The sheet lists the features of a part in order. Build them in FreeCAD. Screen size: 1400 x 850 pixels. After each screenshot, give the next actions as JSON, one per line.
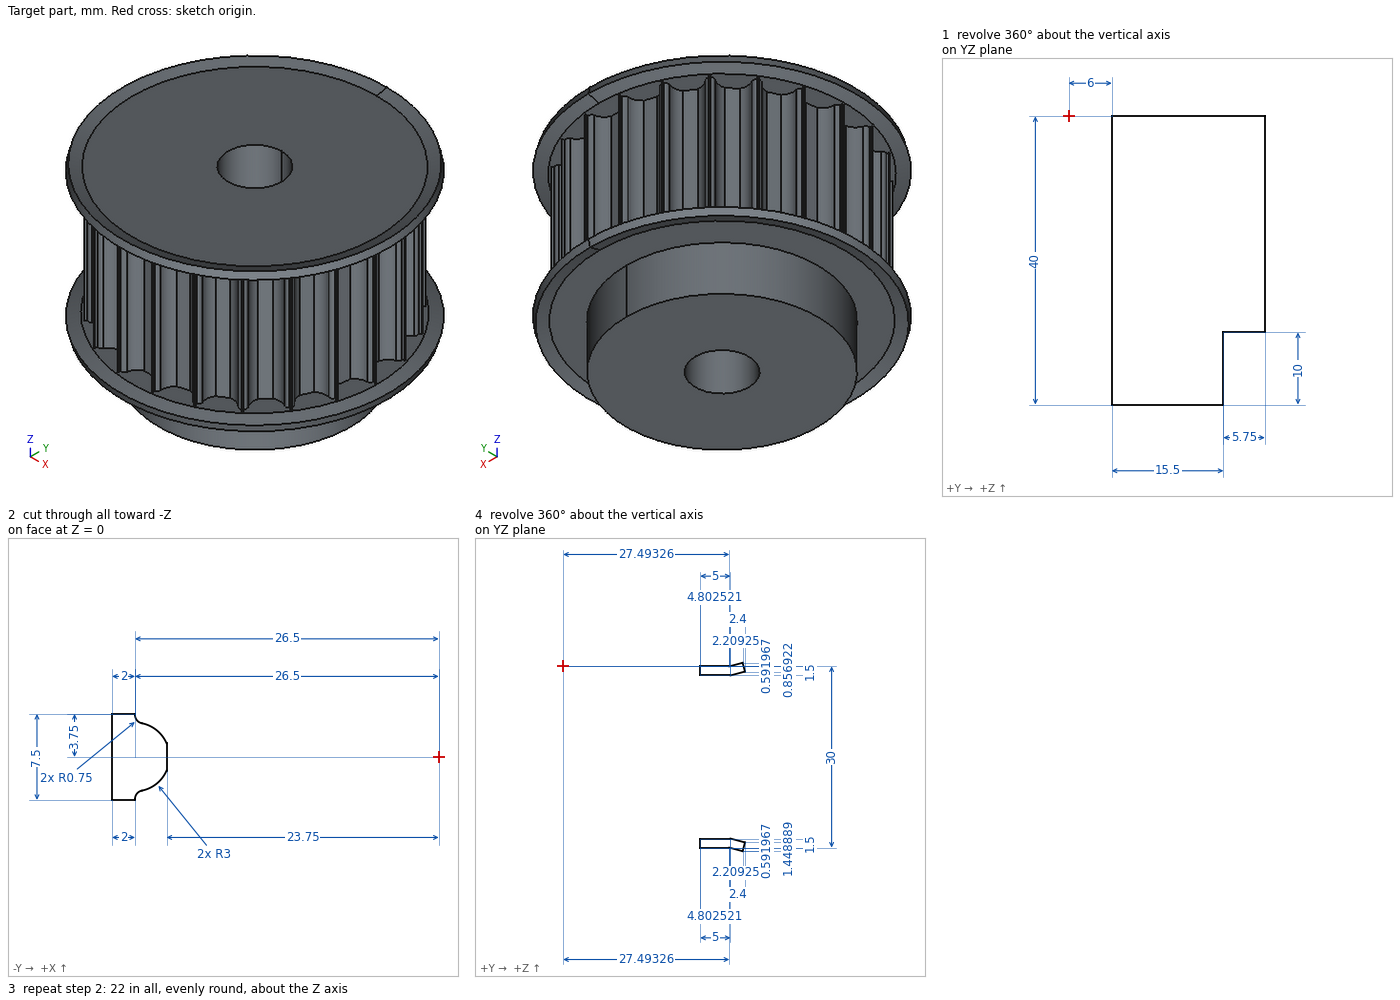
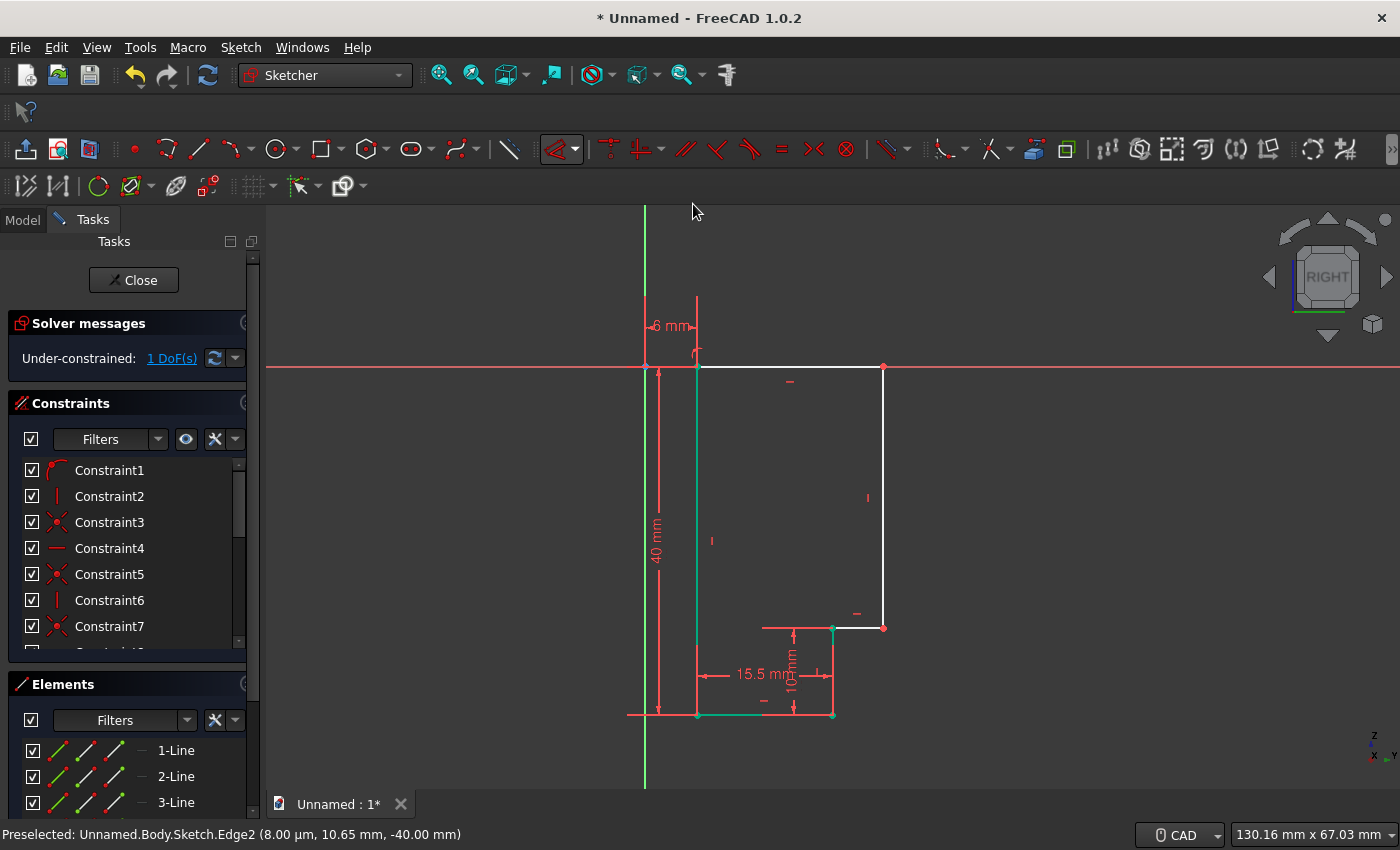
{"action": "left_click", "coordinate": [848, 628]}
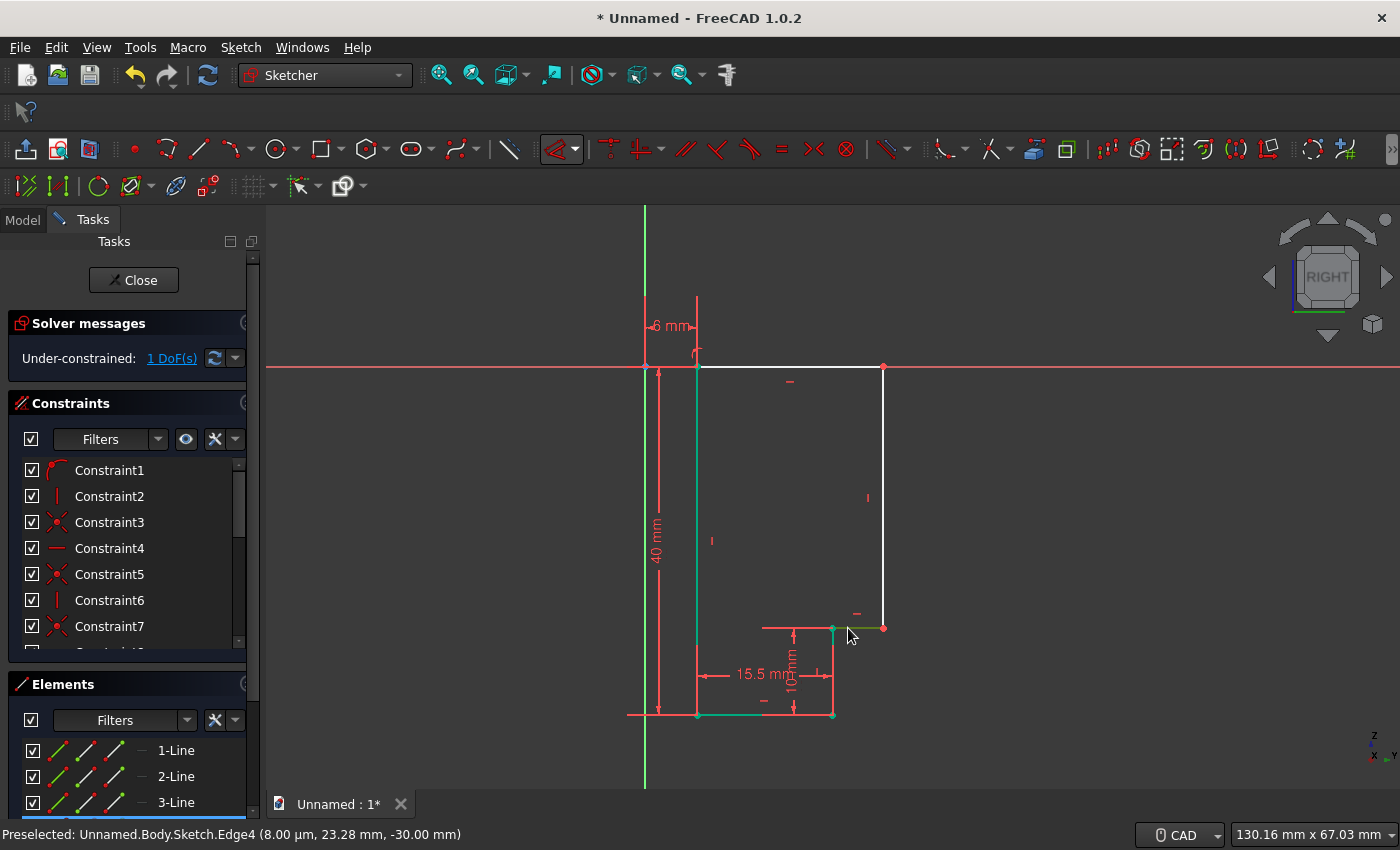
{"action": "key", "text": "l"}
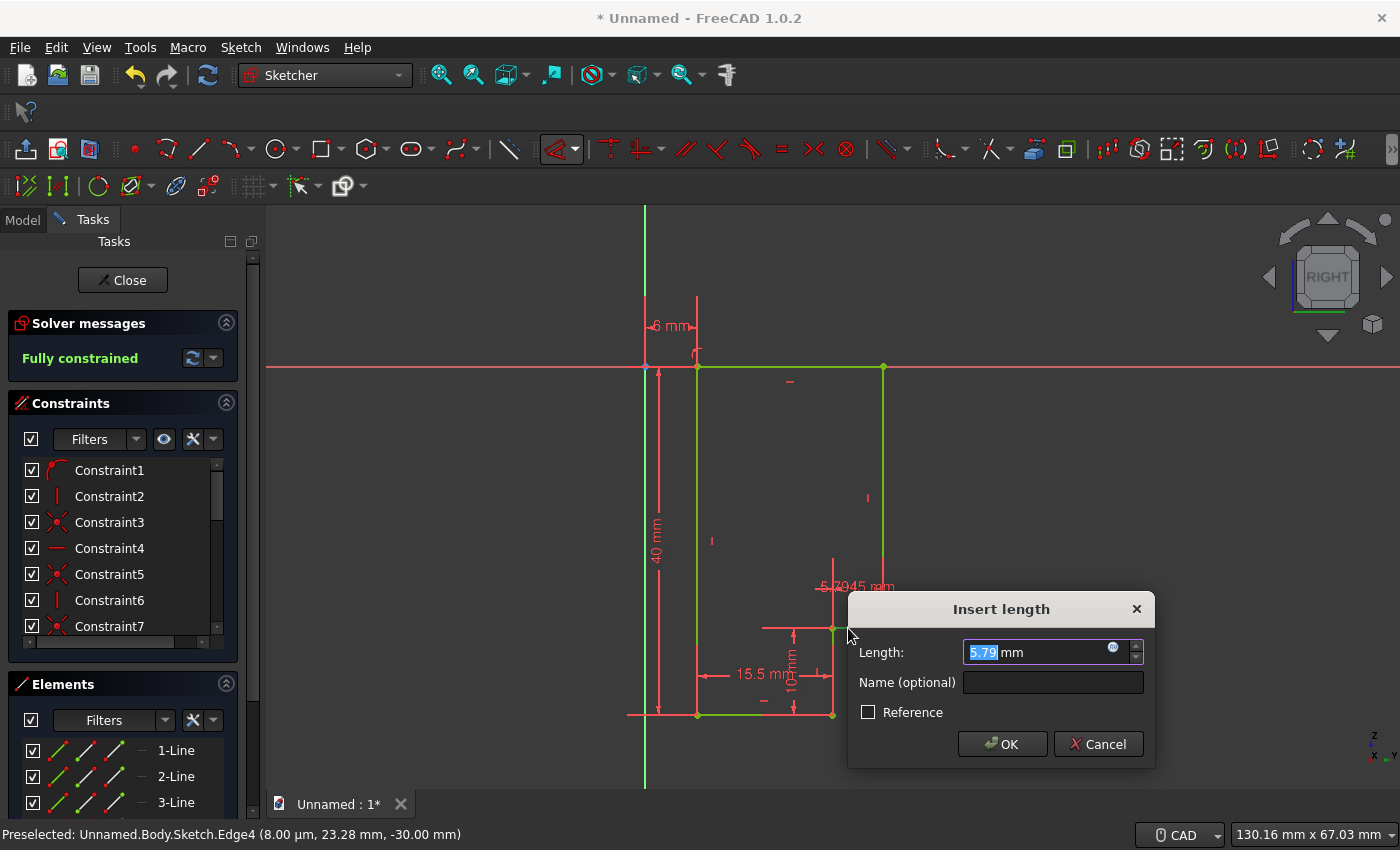
{"action": "type", "text": "5.75"}
{"action": "key", "text": "Return"}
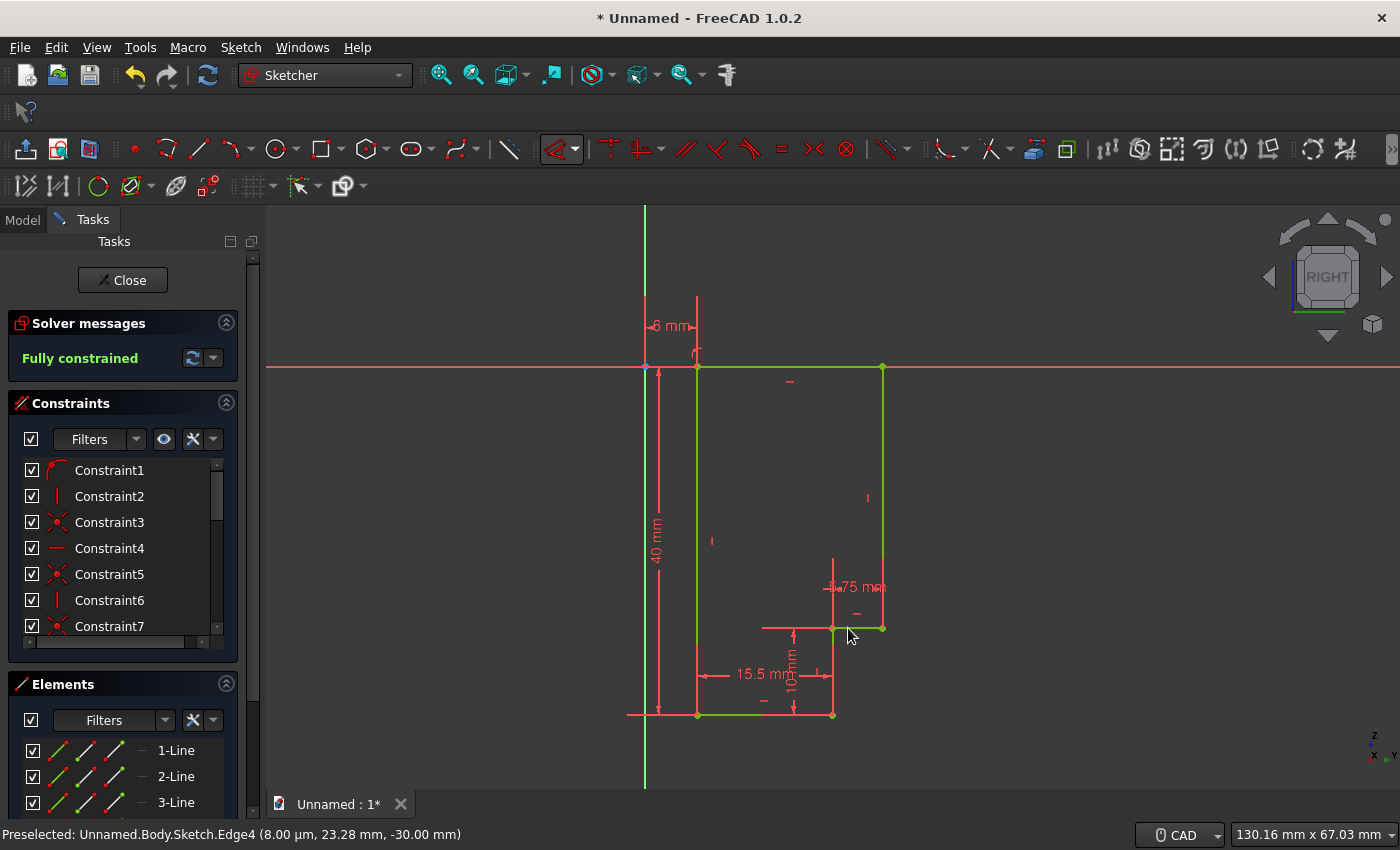
{"action": "left_click", "coordinate": [123, 280]}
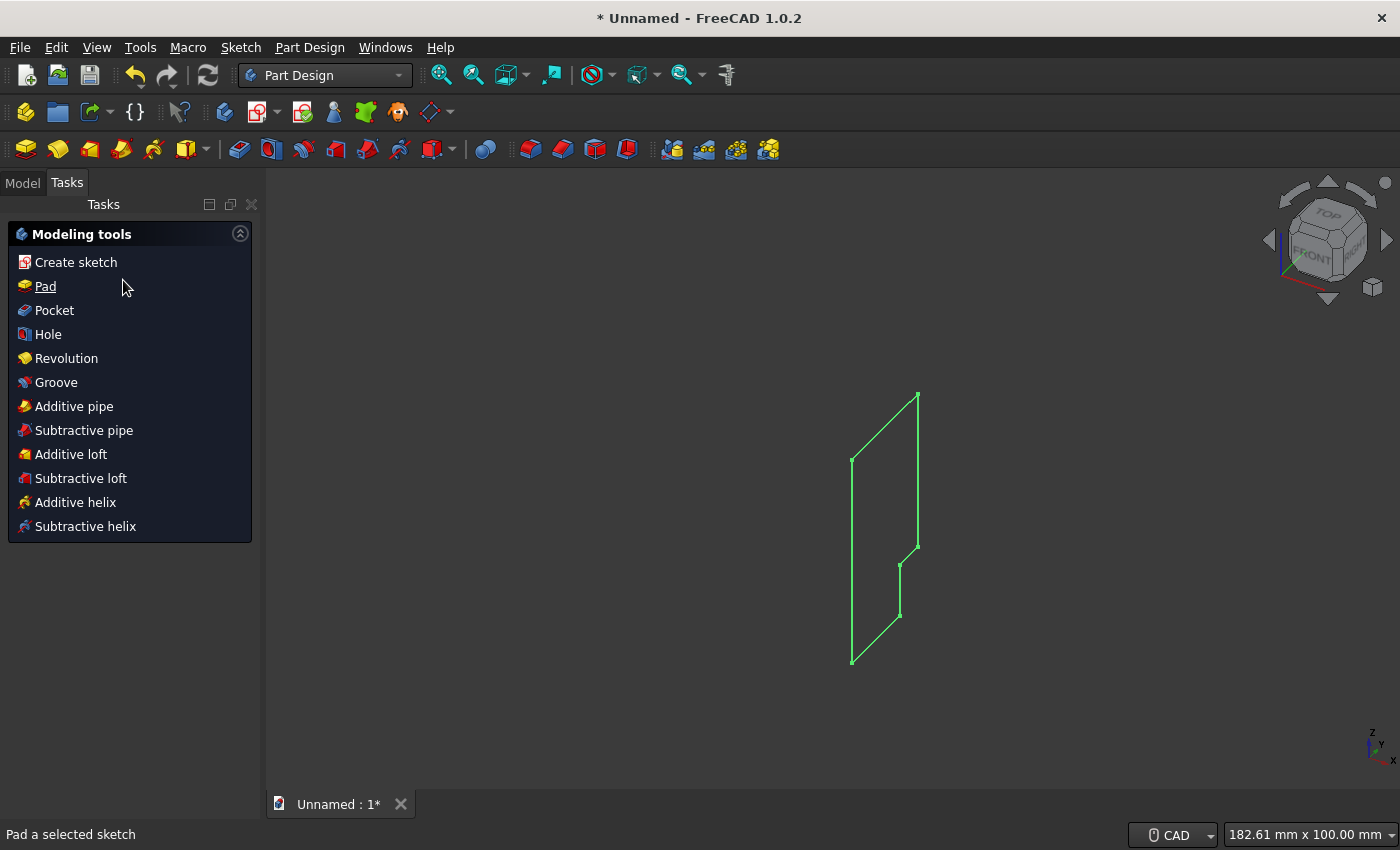
{"action": "left_click", "coordinate": [58, 150]}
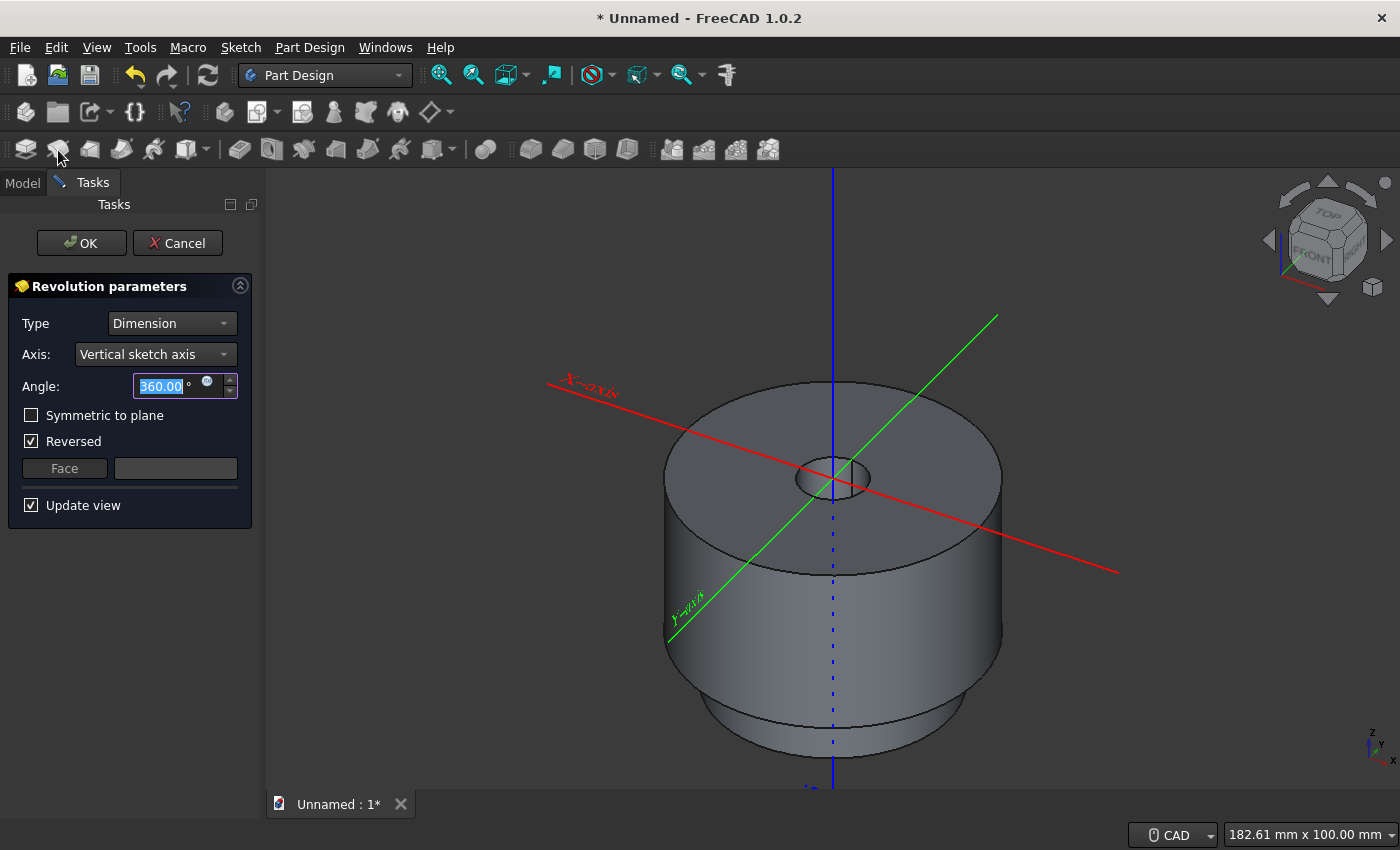
{"action": "left_click", "coordinate": [82, 243]}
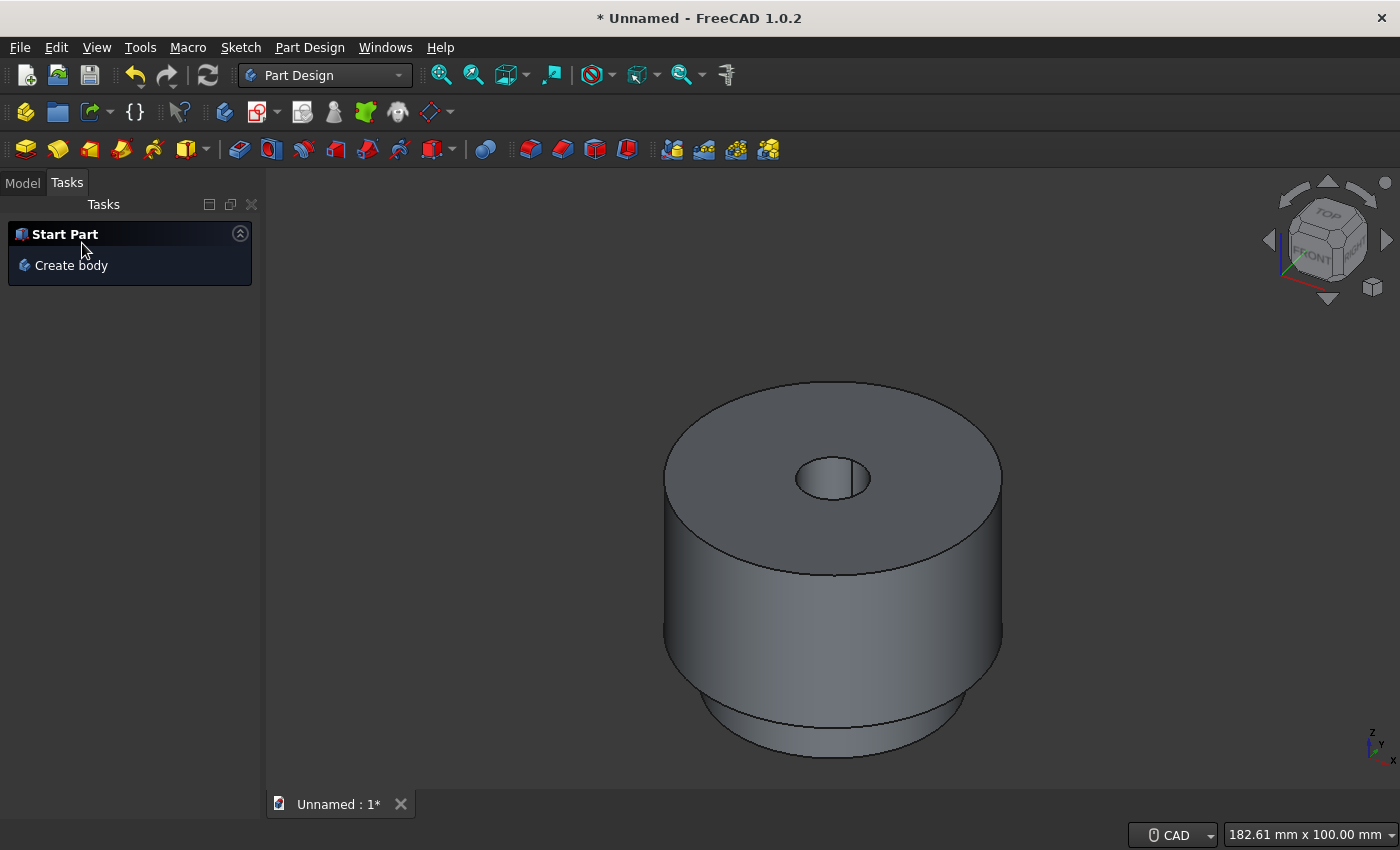
{"action": "left_click", "coordinate": [442, 76]}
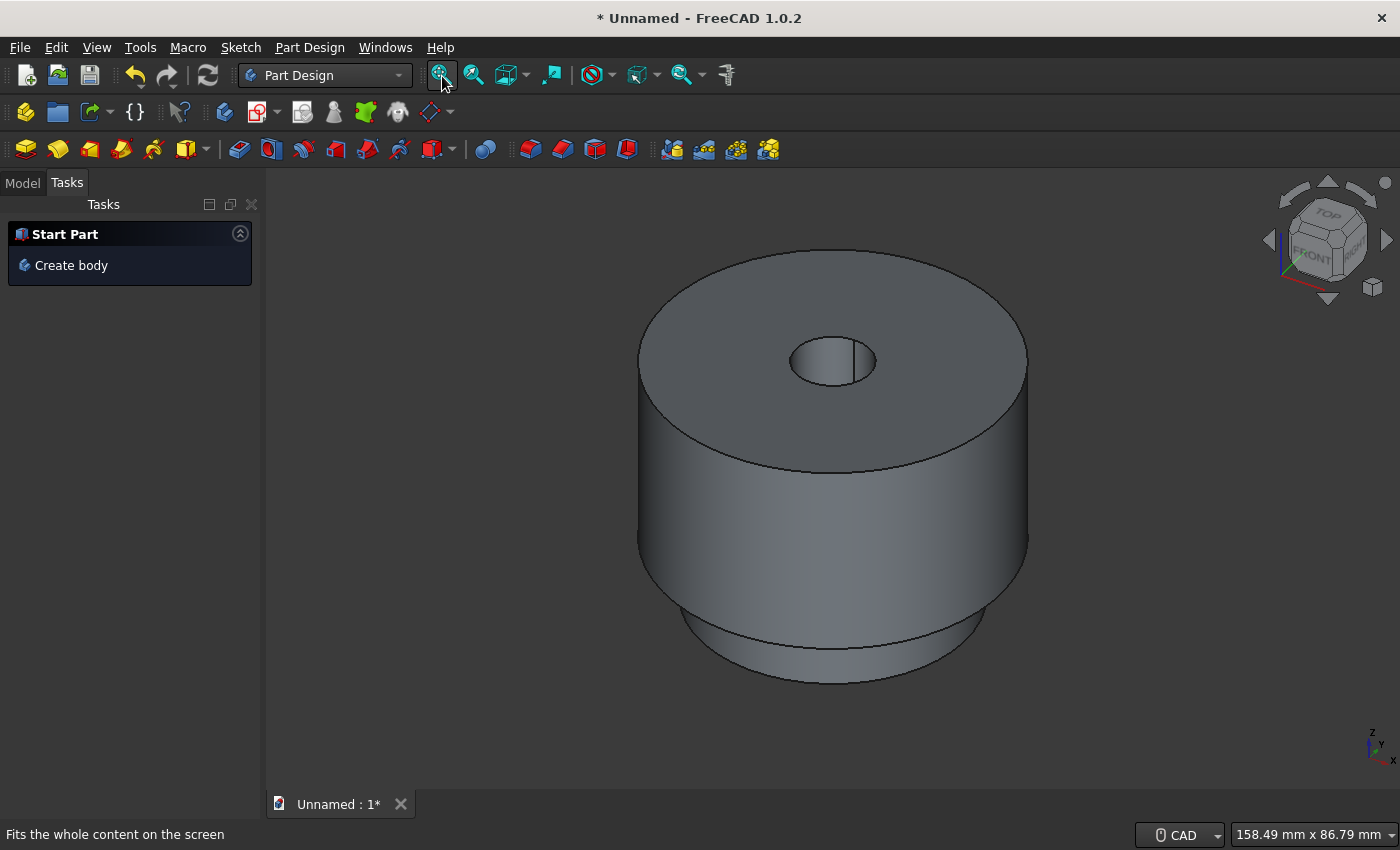
{"action": "left_click", "coordinate": [957, 365]}